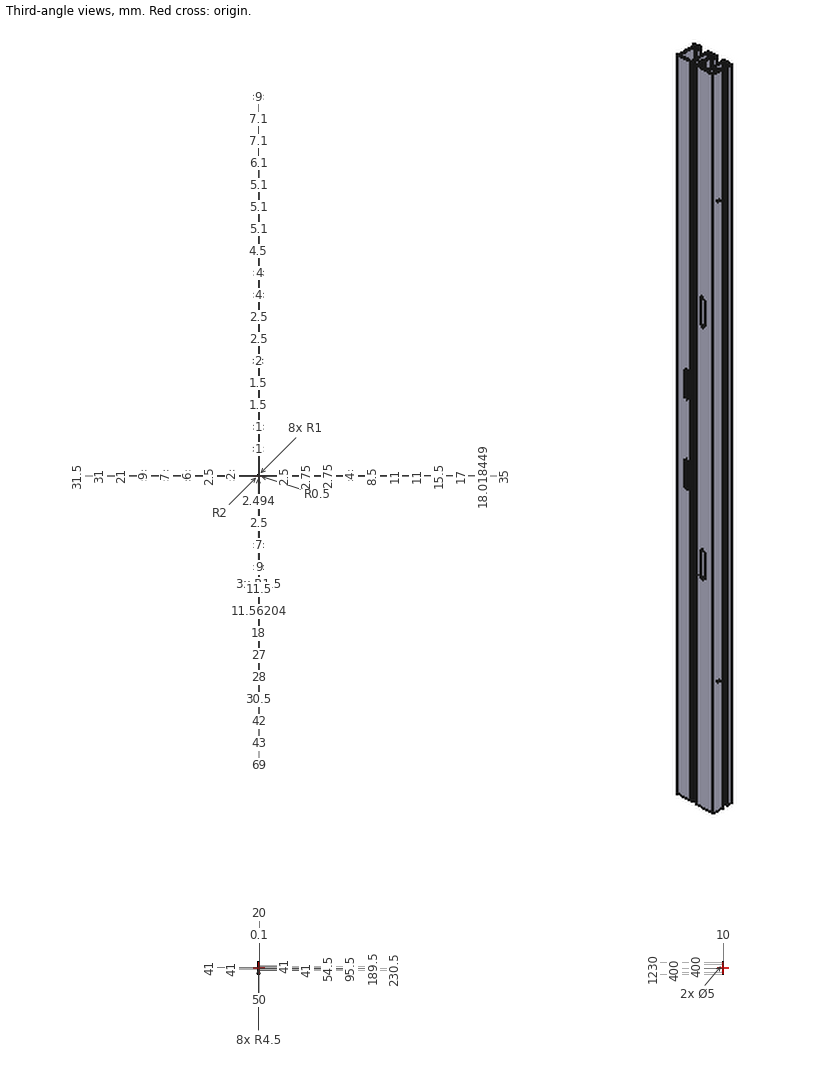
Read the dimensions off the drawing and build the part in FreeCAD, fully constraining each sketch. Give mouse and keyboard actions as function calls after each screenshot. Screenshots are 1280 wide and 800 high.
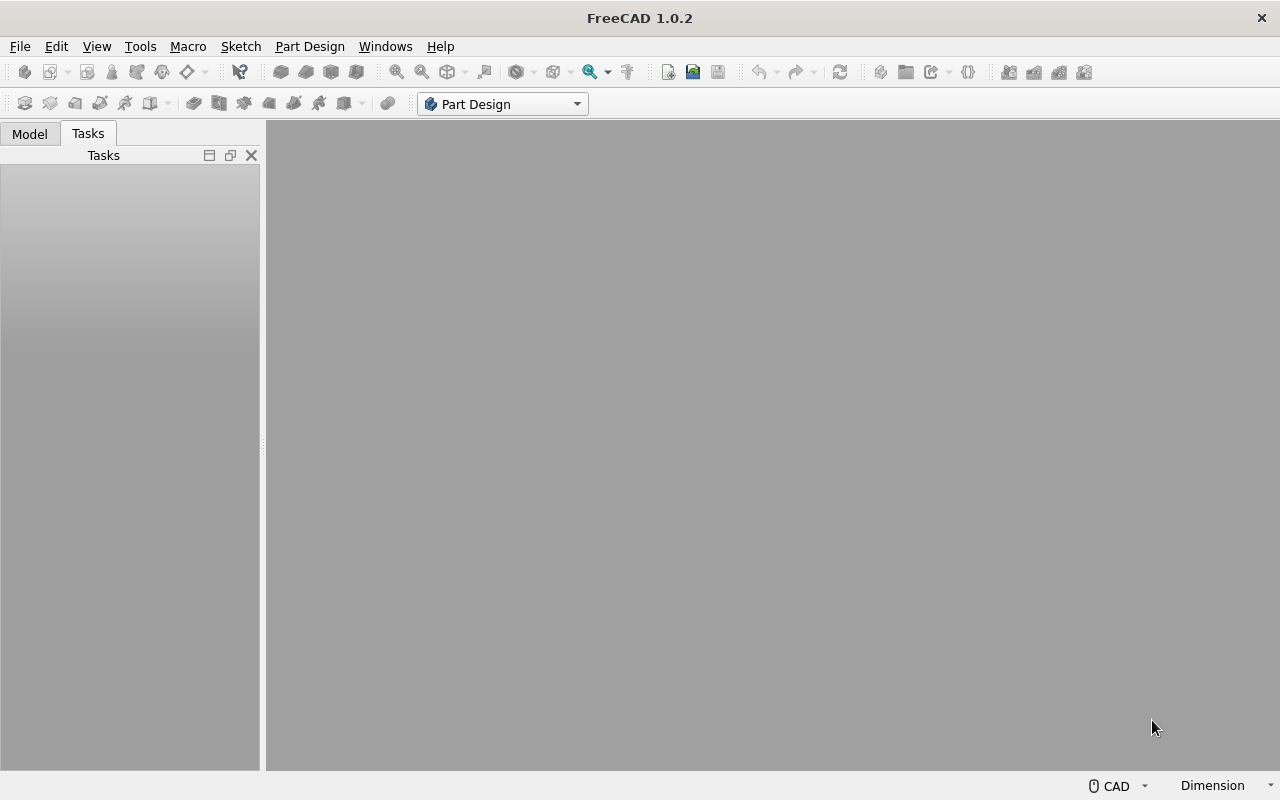
click(668, 72)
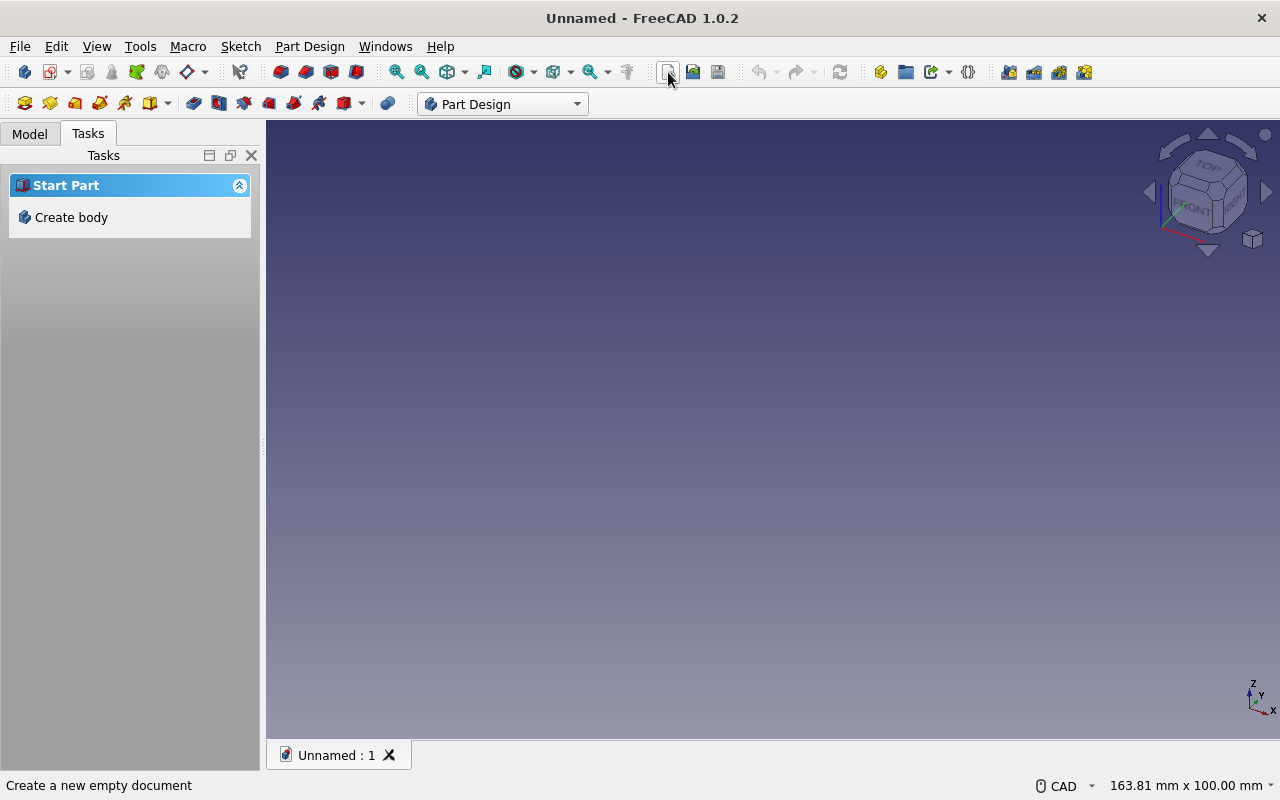
click(50, 72)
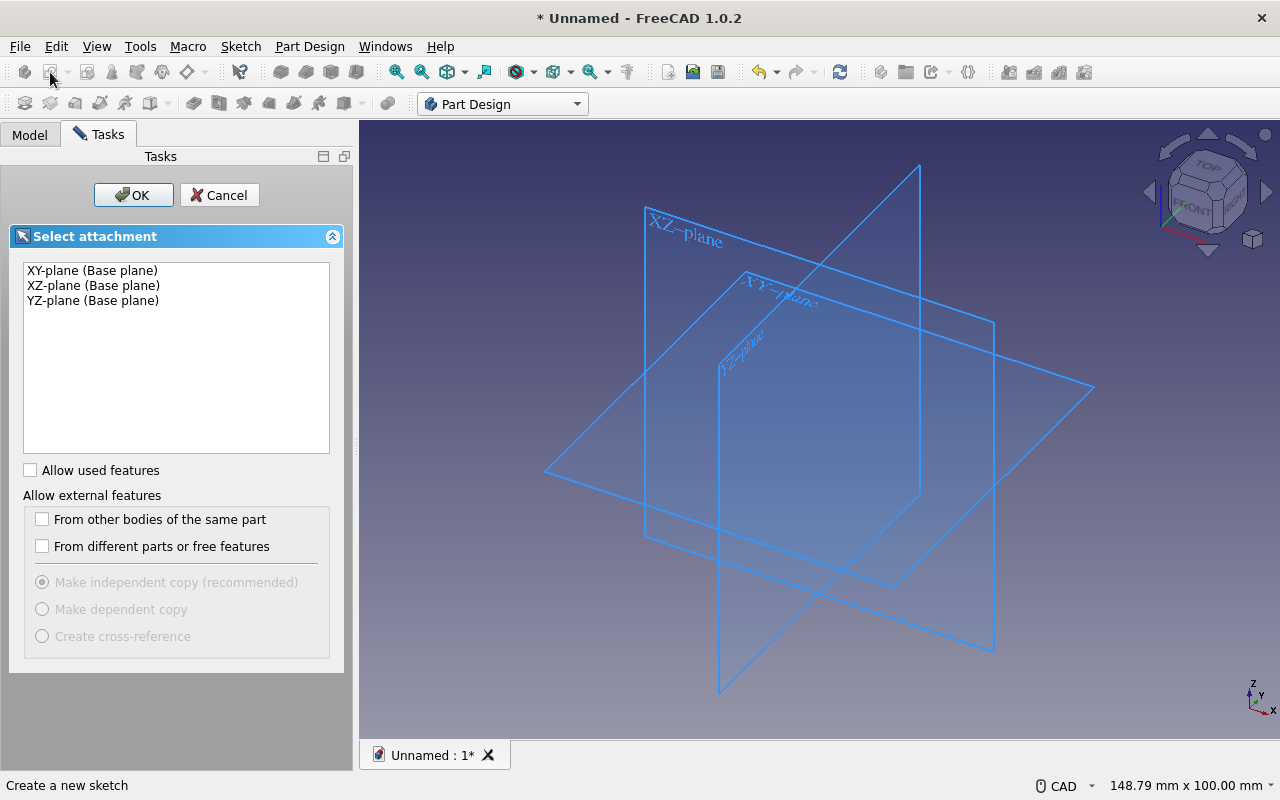
click(84, 270)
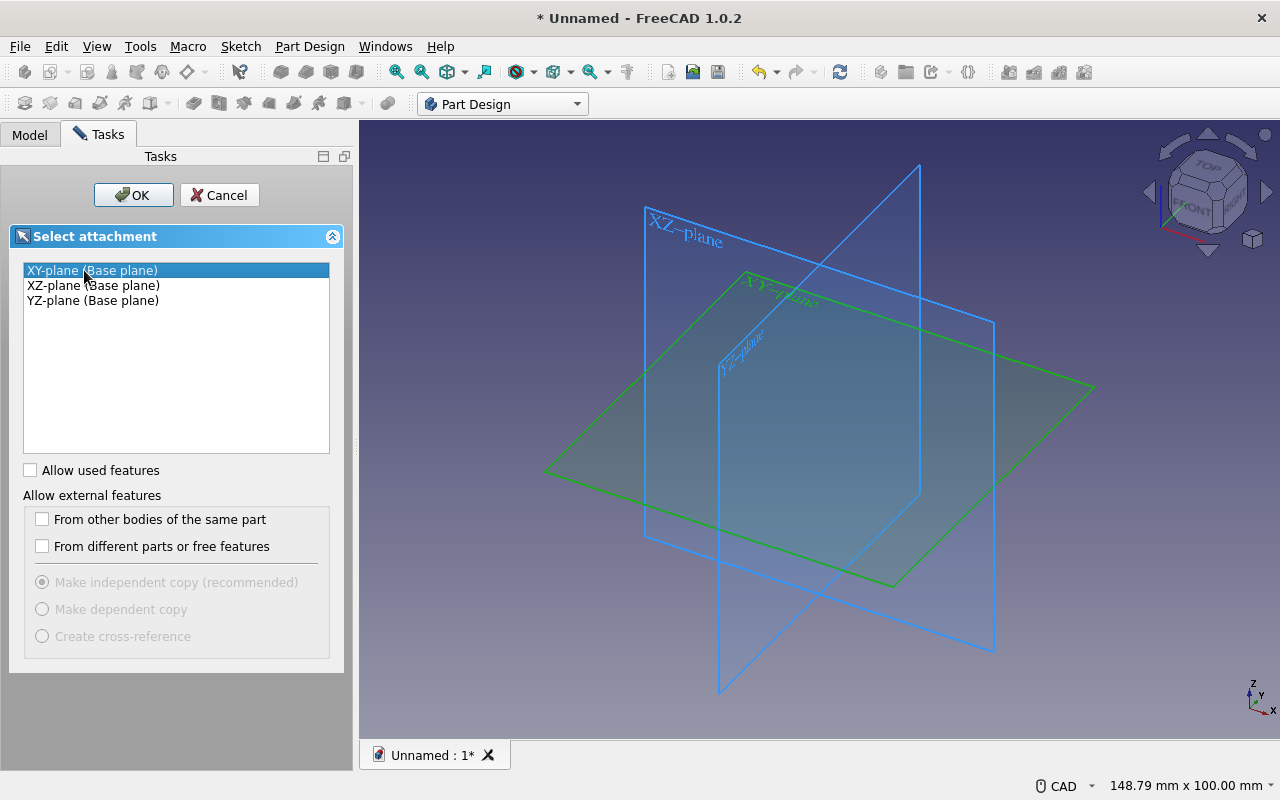
click(134, 195)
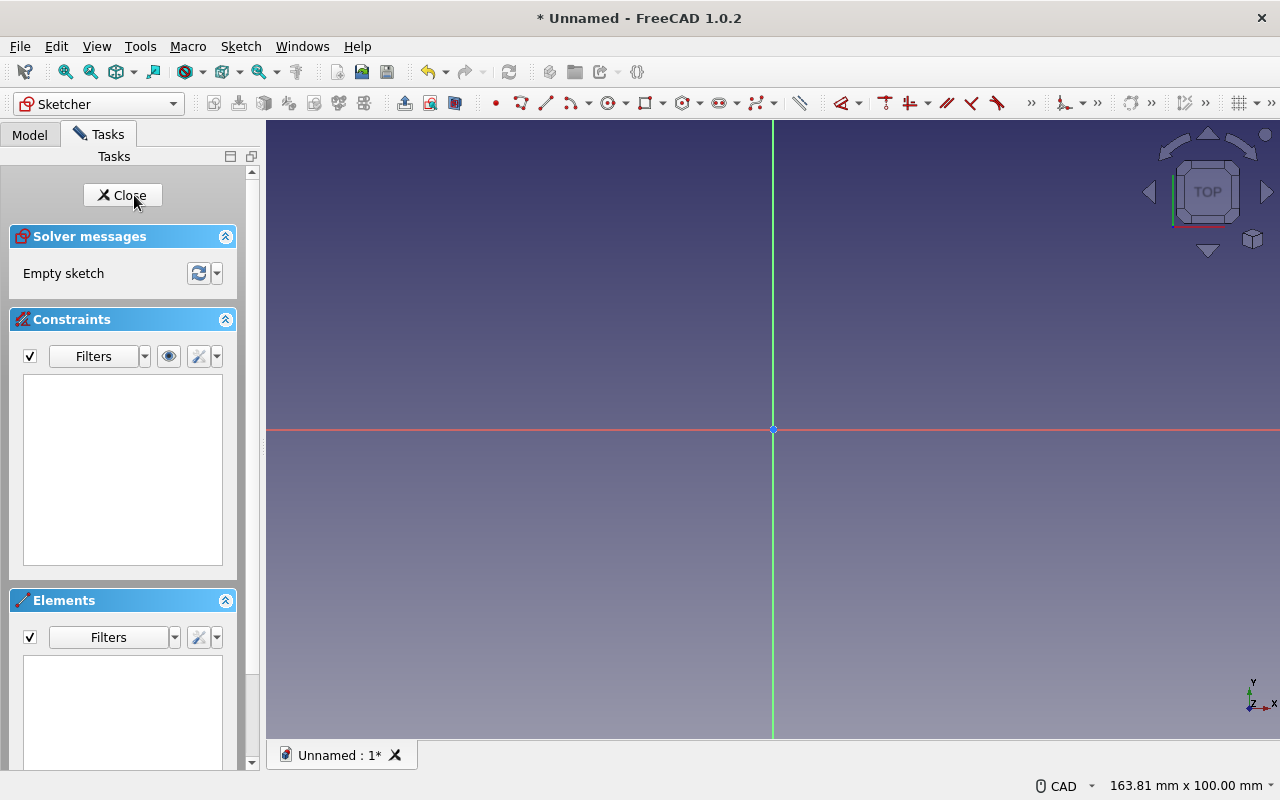
click(546, 104)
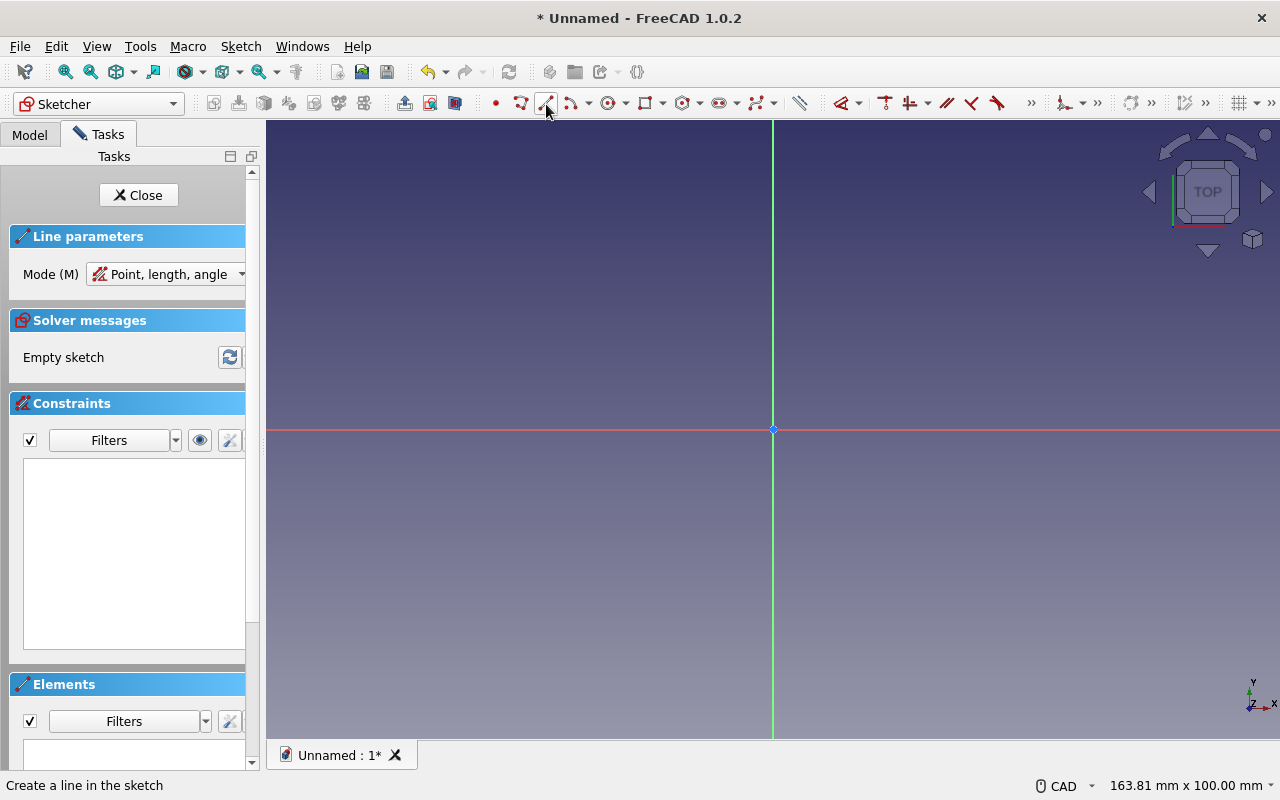
click(606, 213)
click(562, 213)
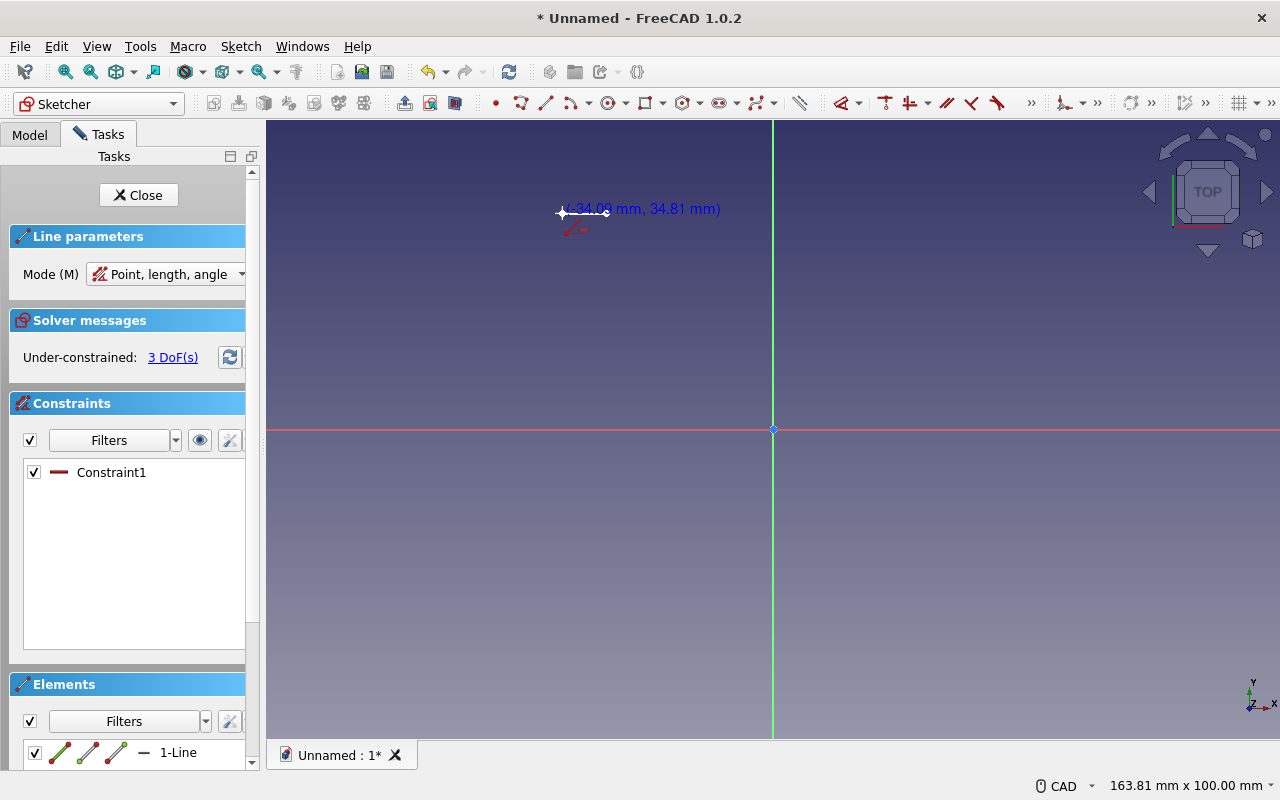
scroll(551, 213, up, 2)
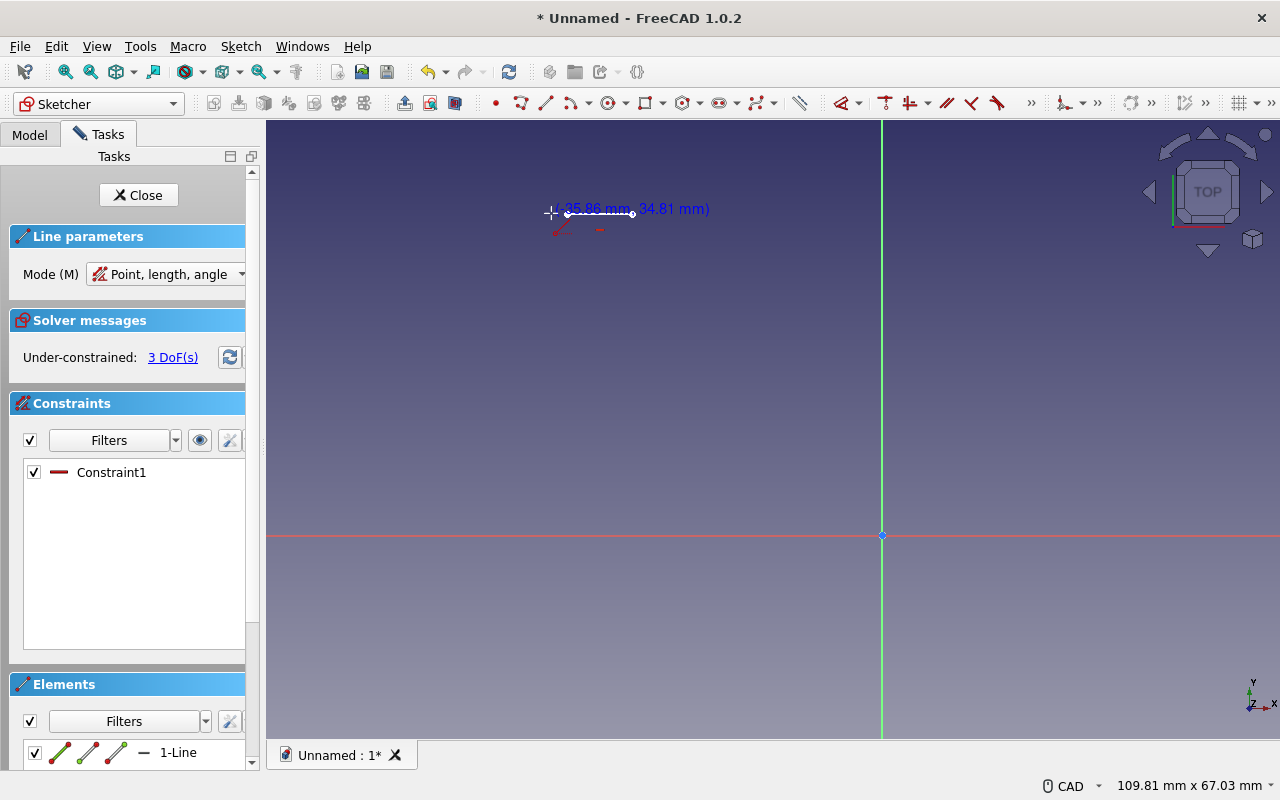
click(551, 213)
click(485, 213)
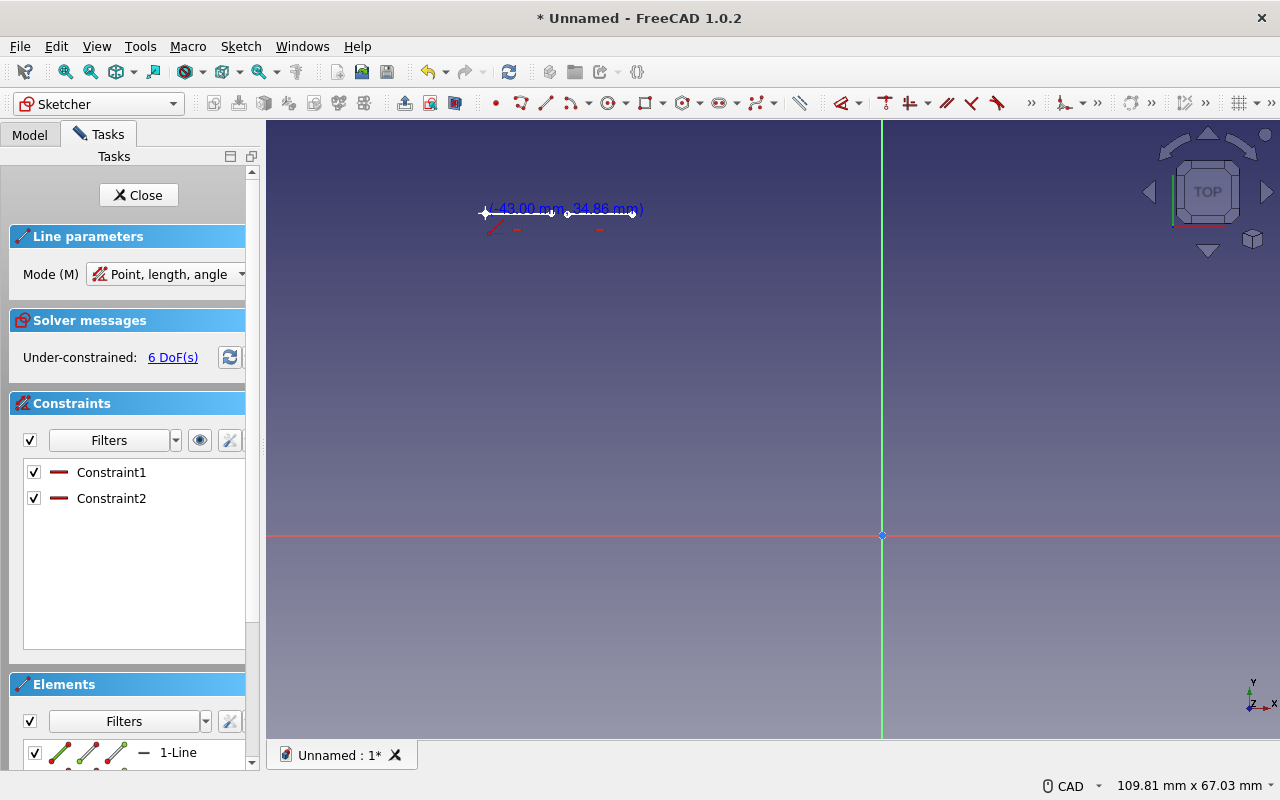
click(521, 104)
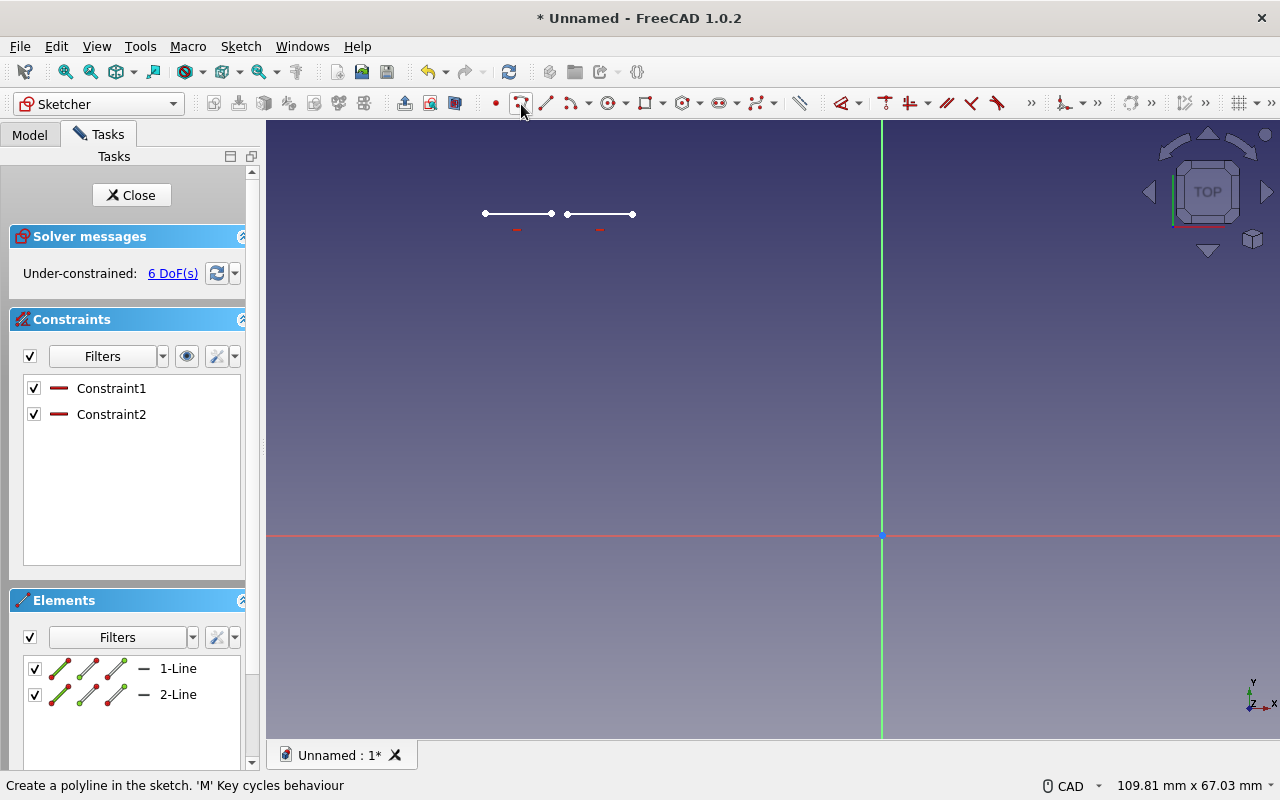
click(476, 222)
click(476, 513)
click(310, 513)
right_click(310, 513)